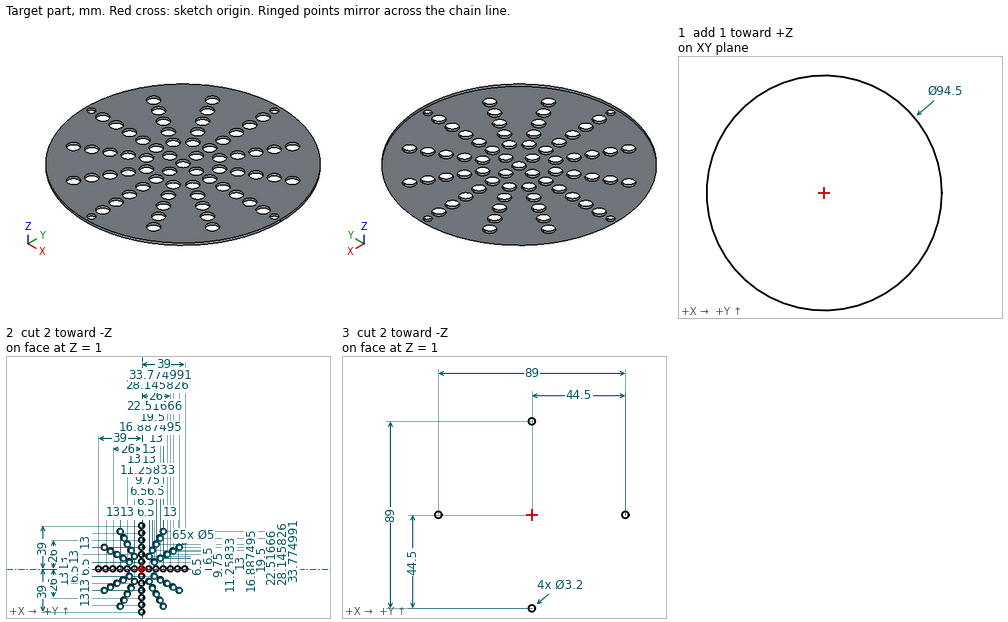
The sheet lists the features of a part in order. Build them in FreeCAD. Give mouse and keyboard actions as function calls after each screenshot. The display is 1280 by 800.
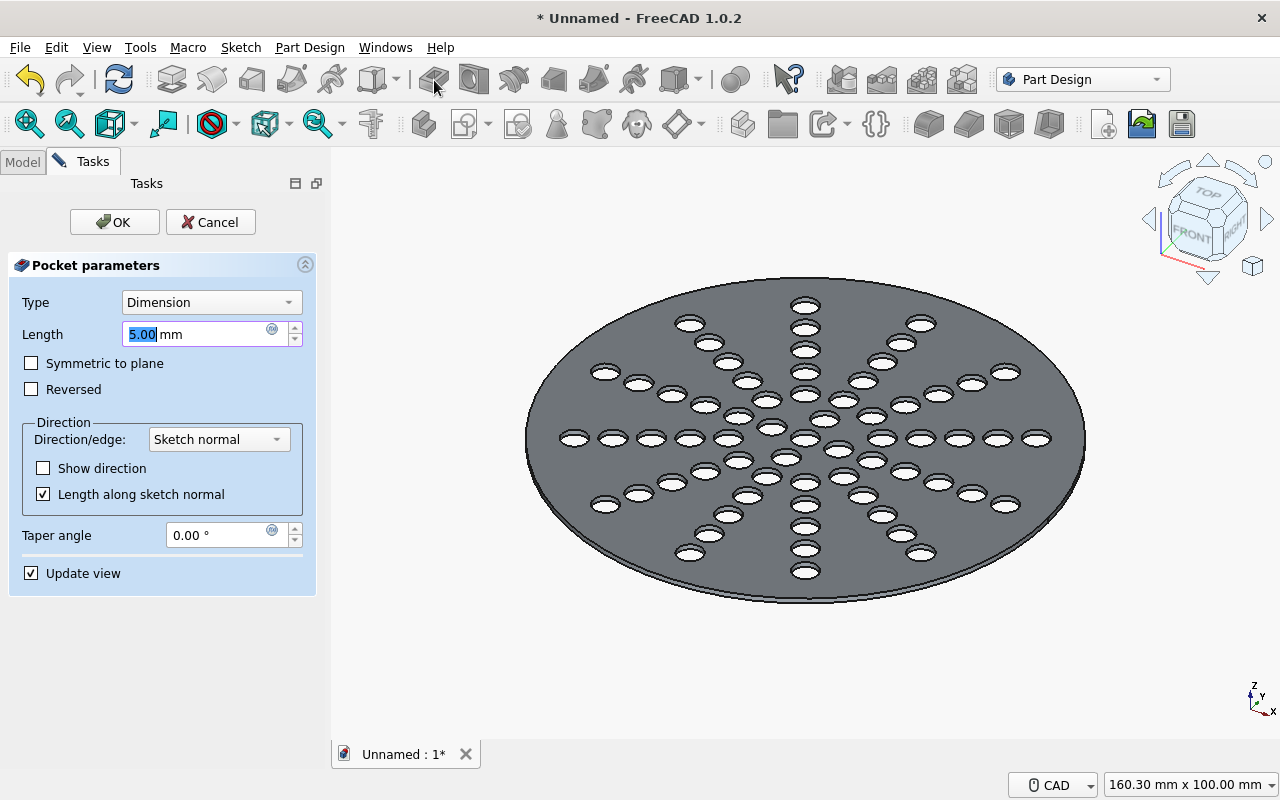
text(2)
key(Tab)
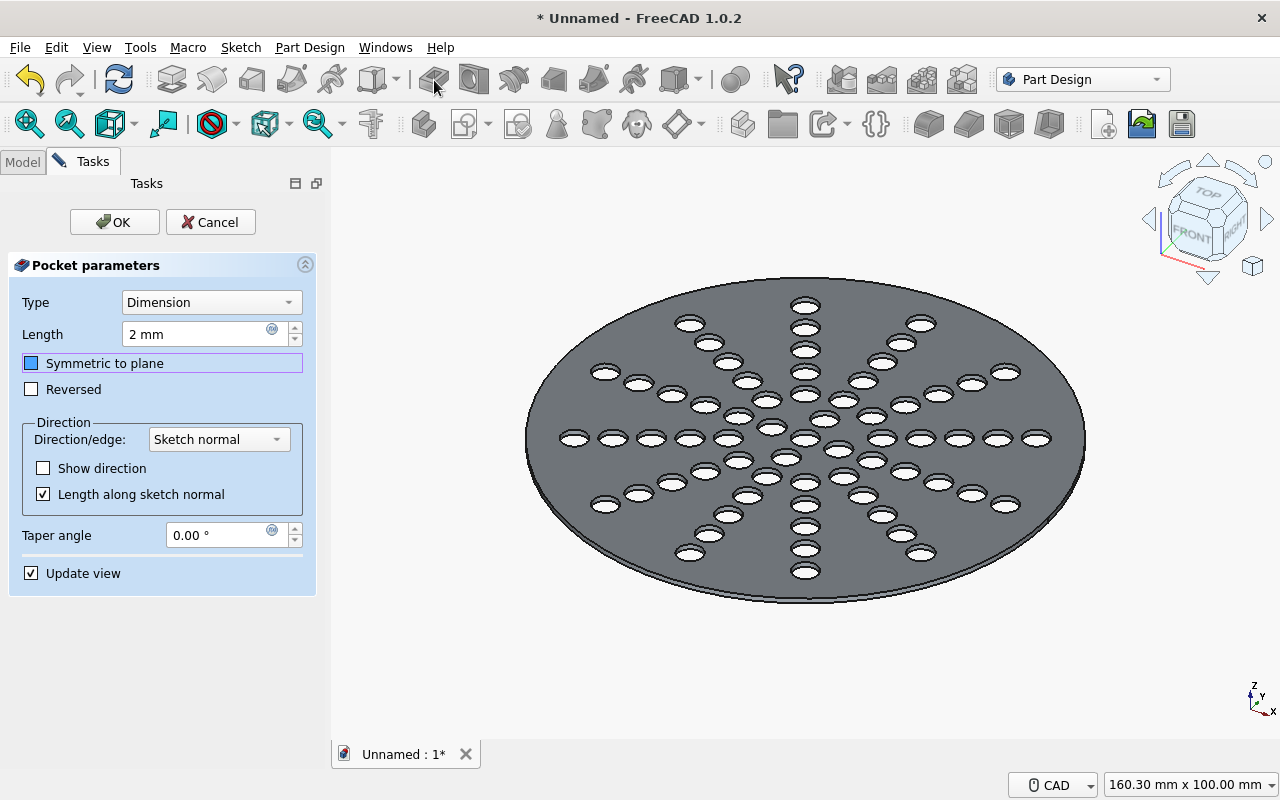
click(115, 222)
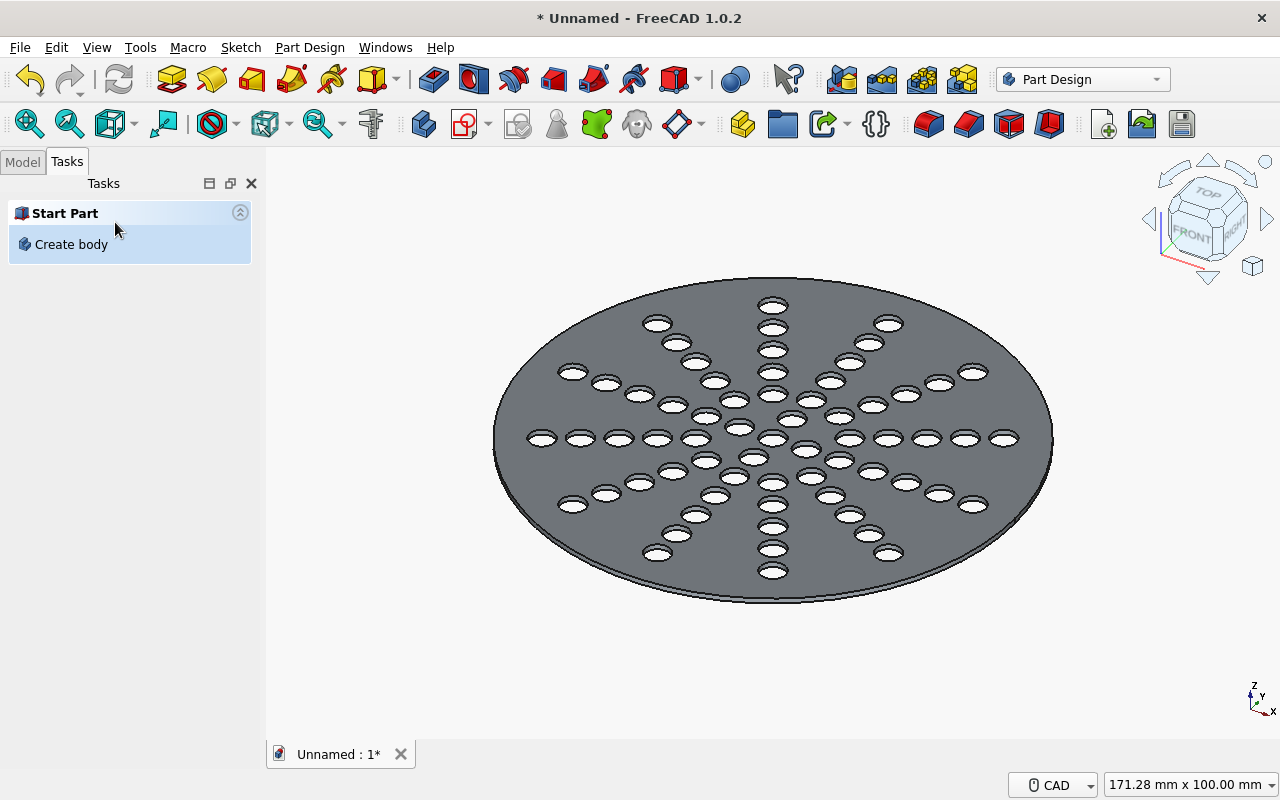
click(714, 312)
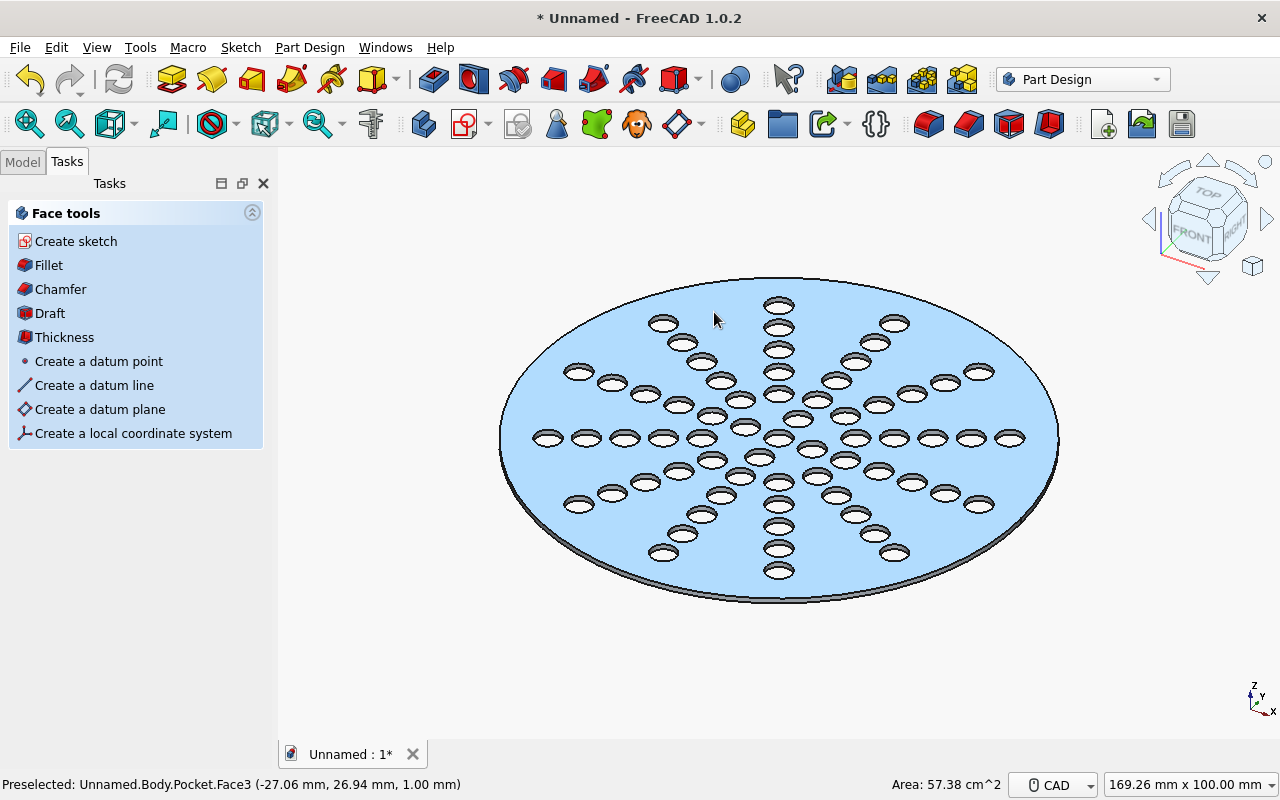
click(464, 124)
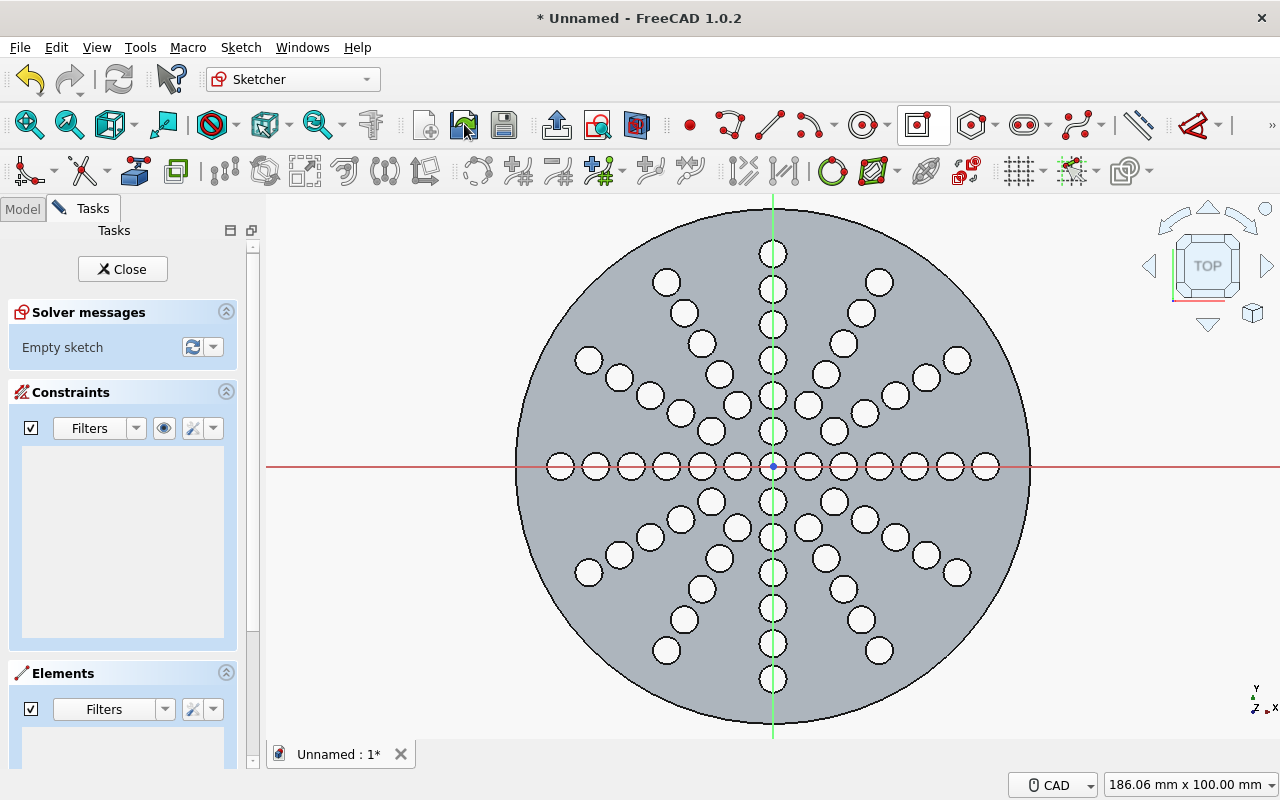
scroll(565, 466, down, 2)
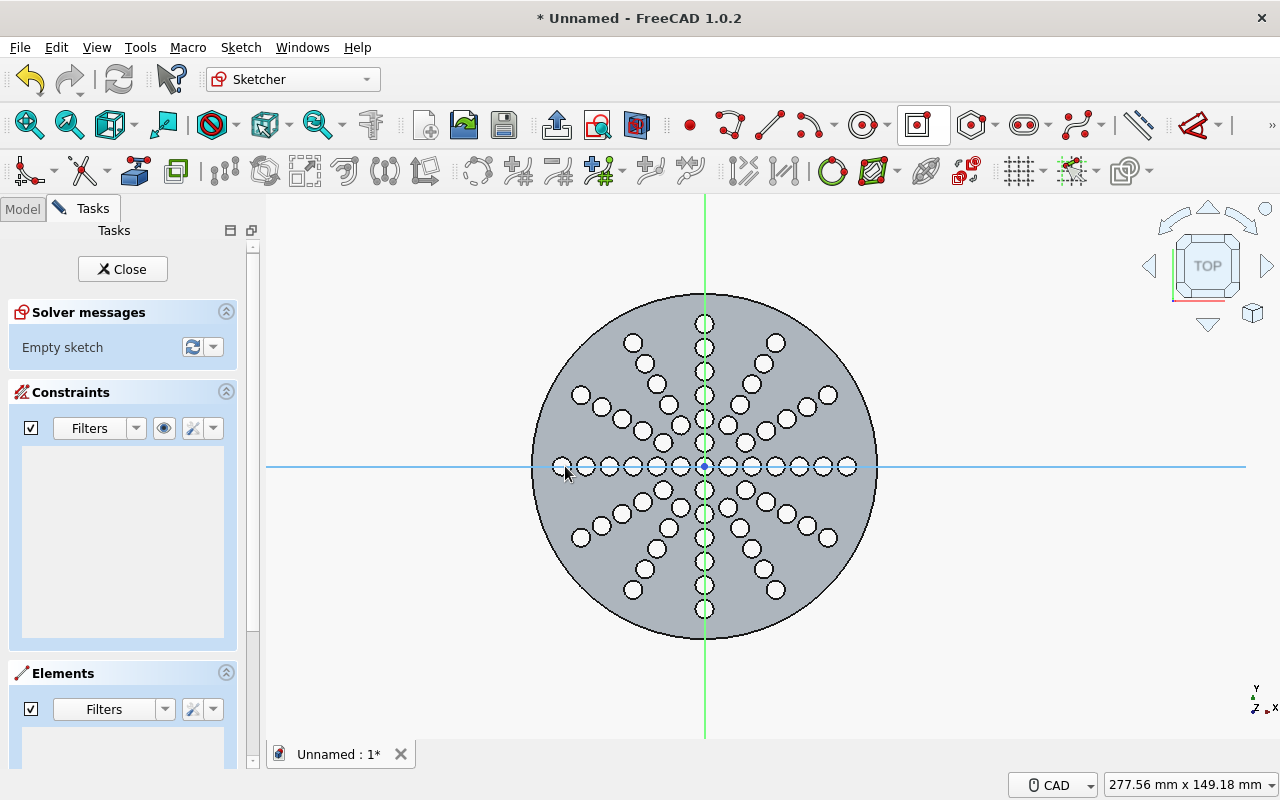
key(g)
key(c)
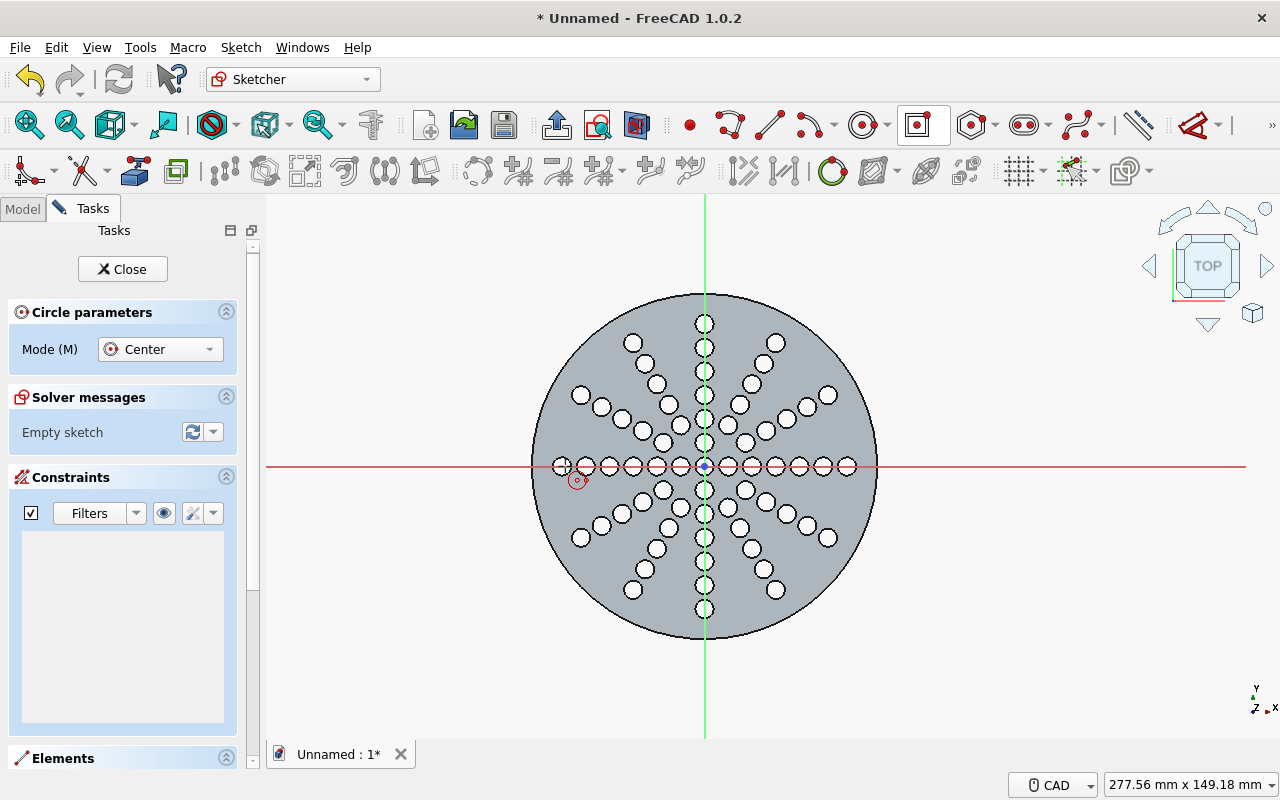
scroll(705, 629, up, 7)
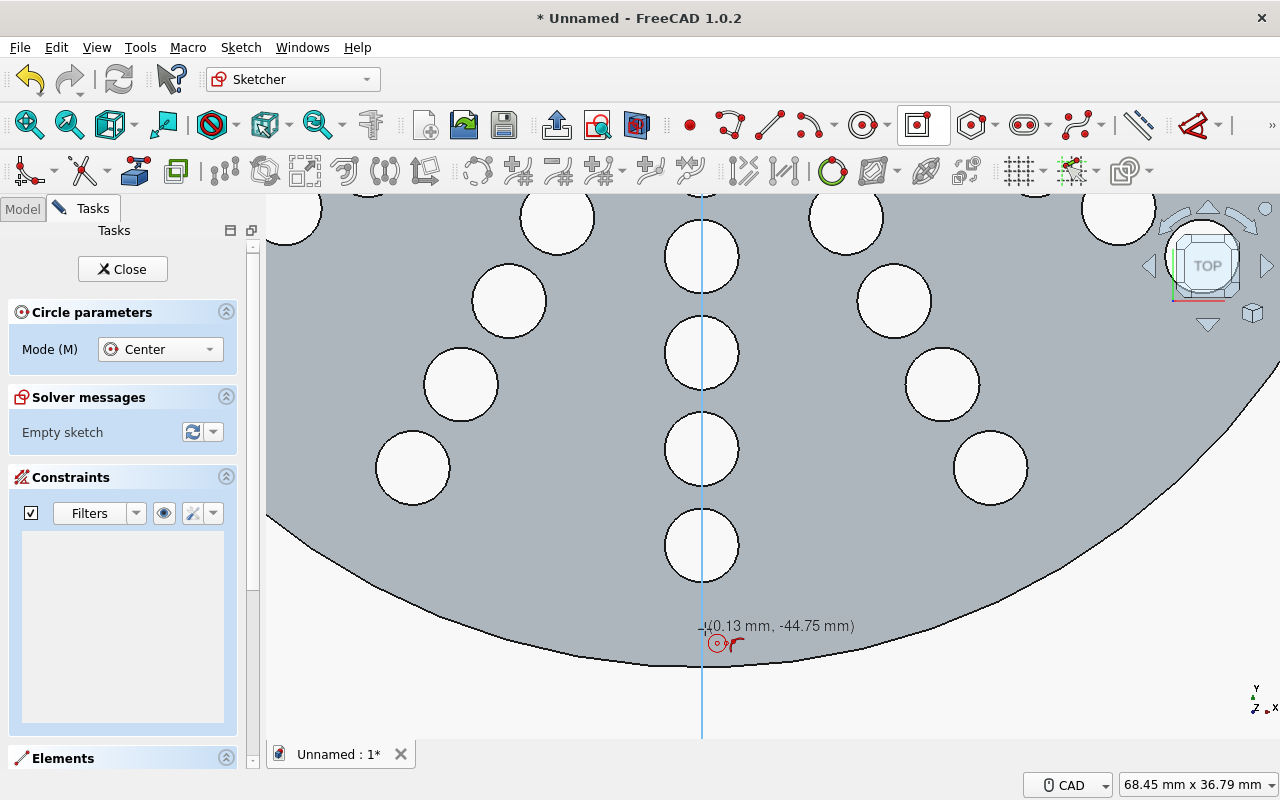
scroll(705, 630, down, 7)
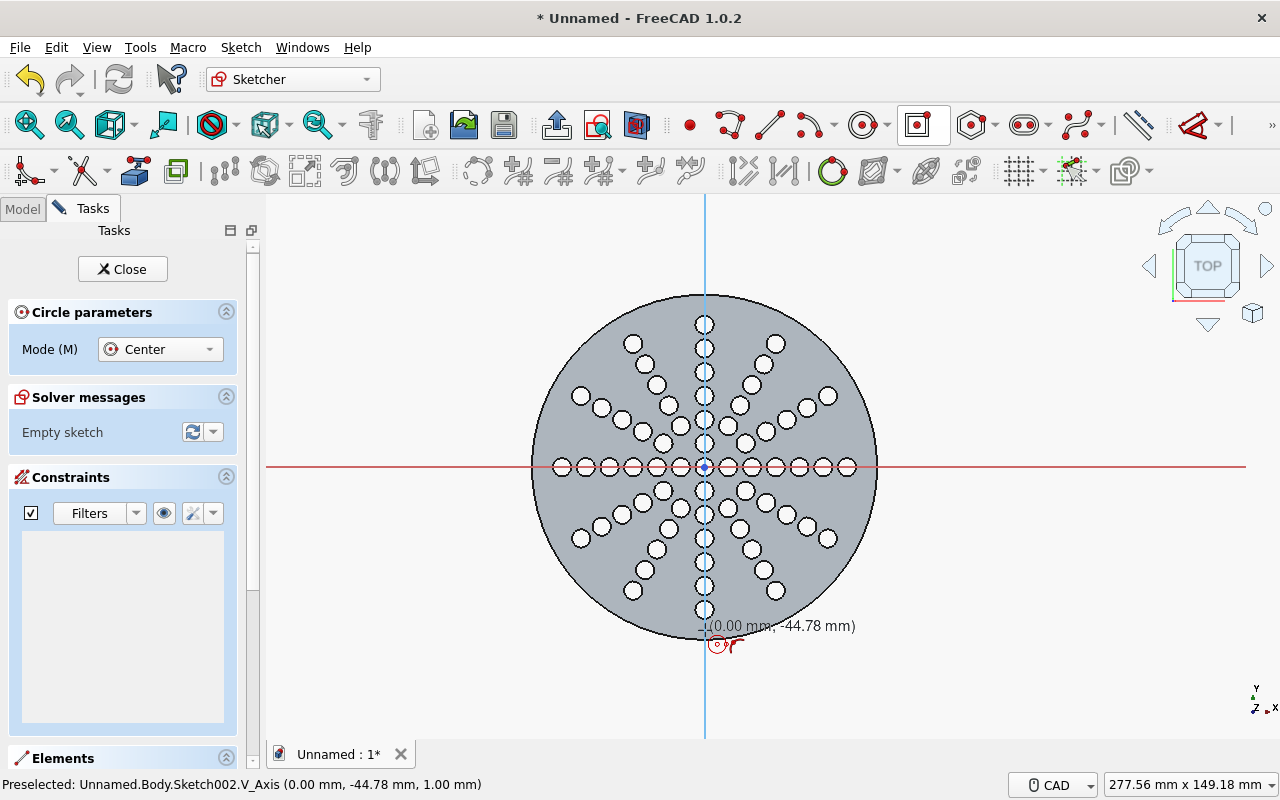
click(705, 630)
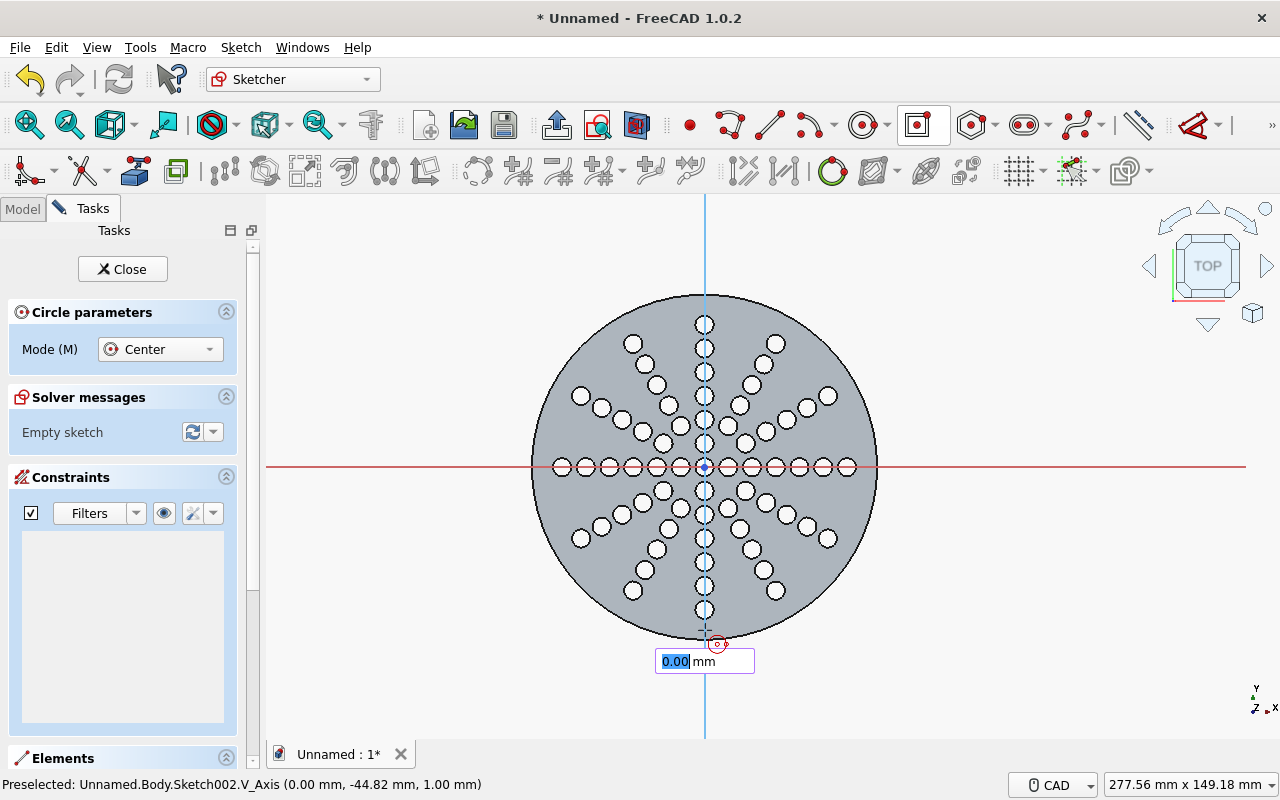
scroll(710, 628, up, 6)
move(709, 626)